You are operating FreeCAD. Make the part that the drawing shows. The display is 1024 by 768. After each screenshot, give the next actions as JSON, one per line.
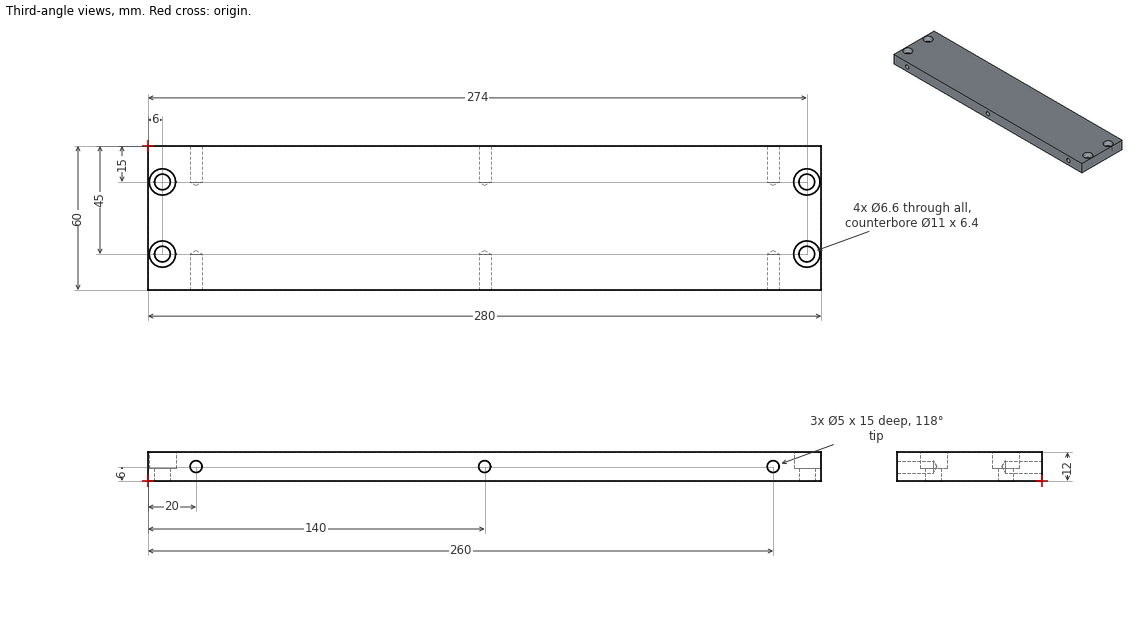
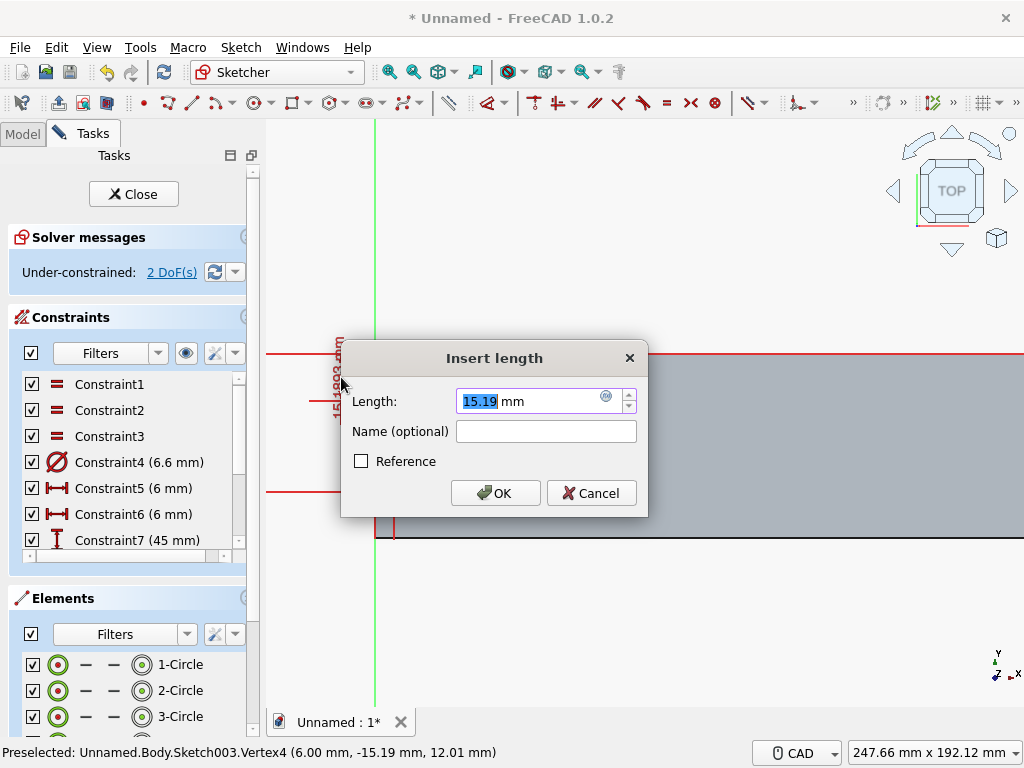
{"action": "type", "text": "15"}
{"action": "key", "text": "Return"}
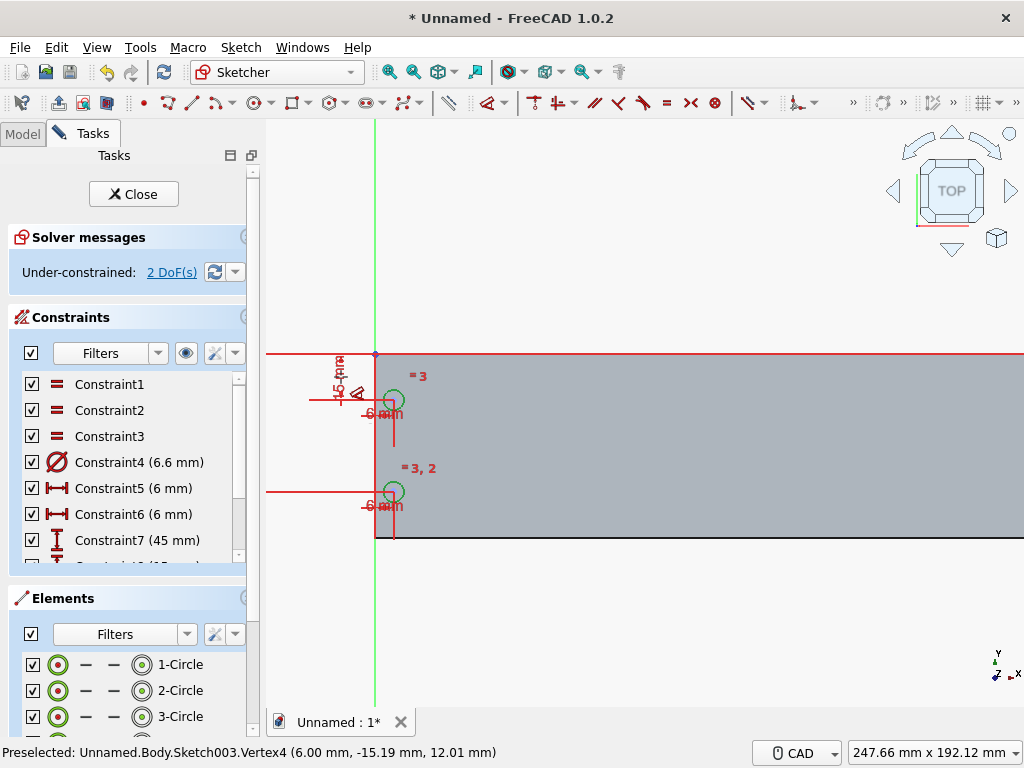
{"action": "scroll", "coordinate": [394, 401], "scroll_direction": "down", "scroll_amount": 4}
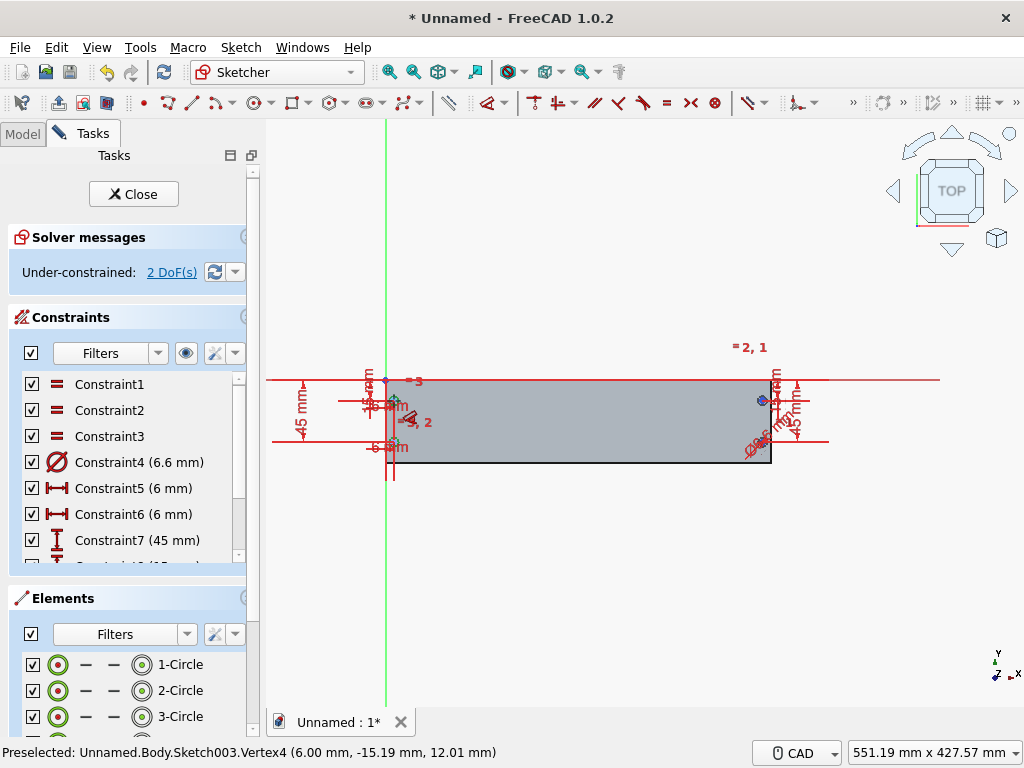
{"action": "left_click", "coordinate": [763, 442]}
{"action": "left_click", "coordinate": [574, 346]}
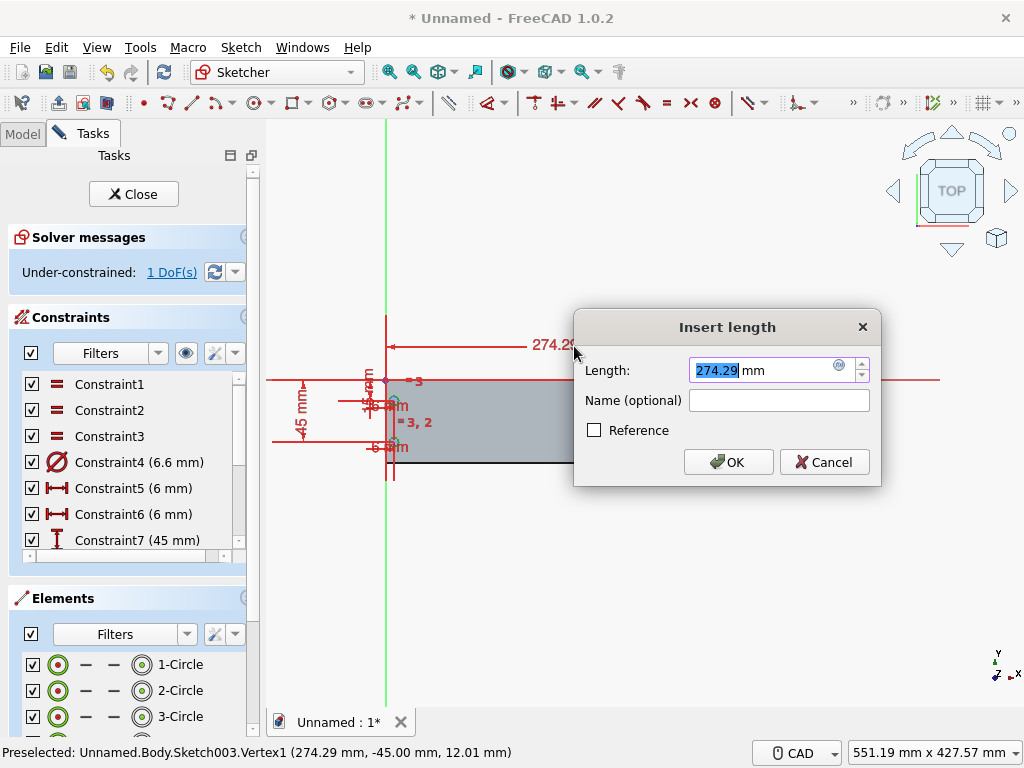
{"action": "type", "text": "274"}
{"action": "key", "text": "Return"}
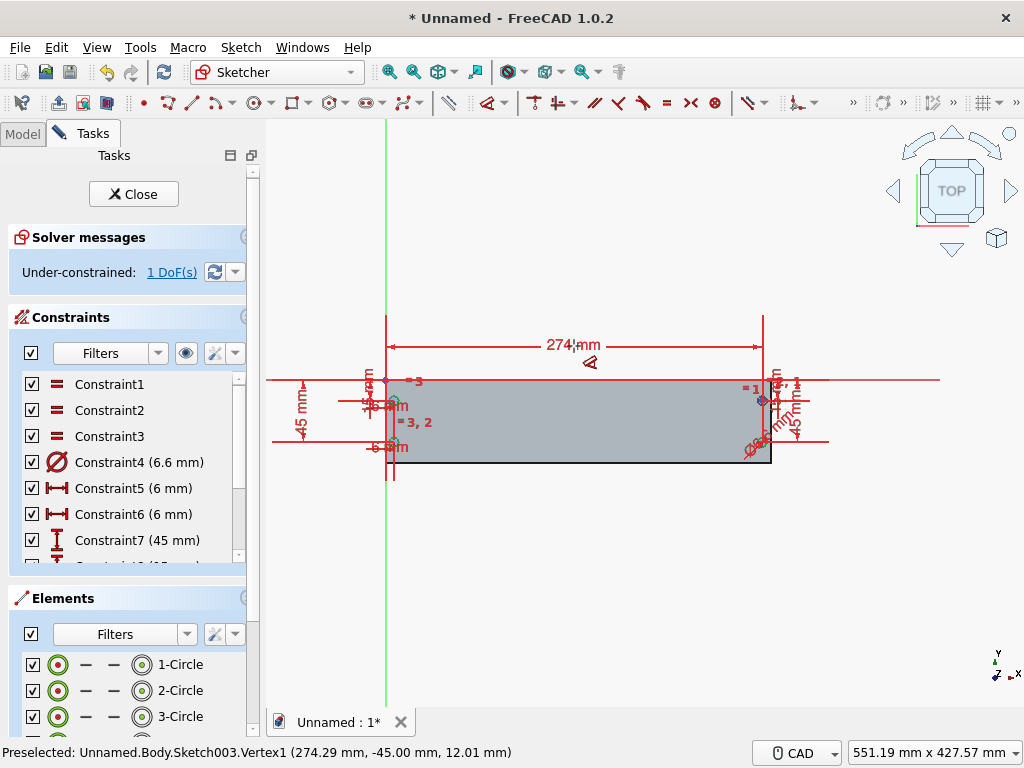
{"action": "left_click", "coordinate": [762, 401]}
{"action": "left_click", "coordinate": [487, 346]}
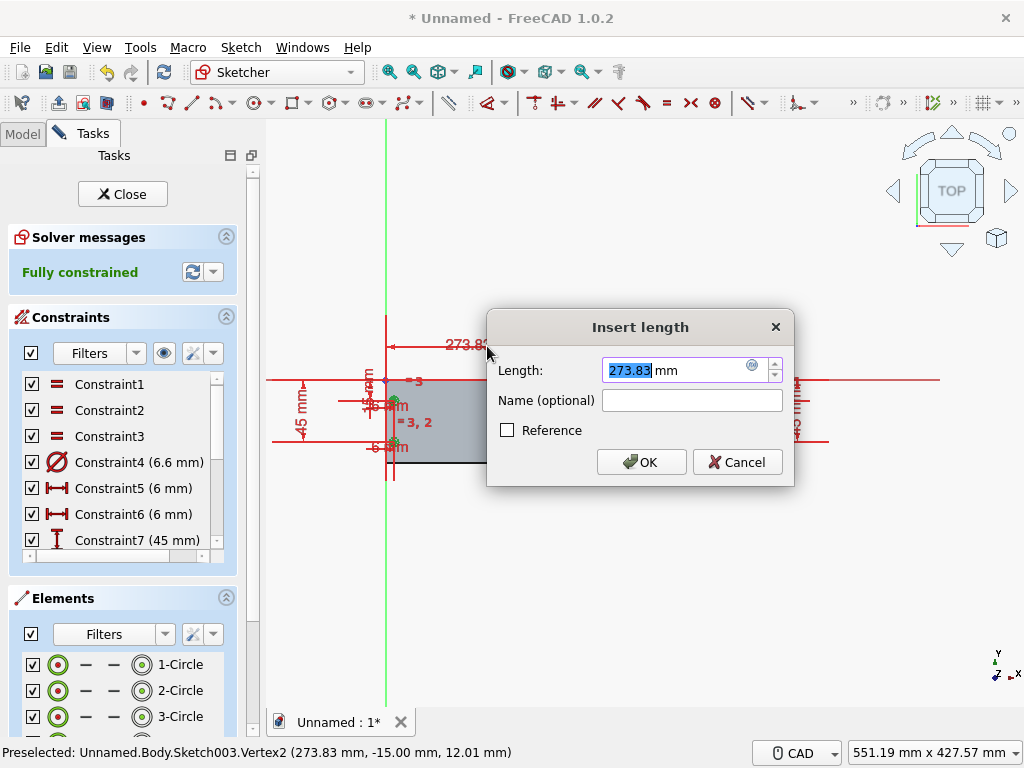
{"action": "type", "text": "274"}
{"action": "key", "text": "Return"}
{"action": "key", "text": "Escape"}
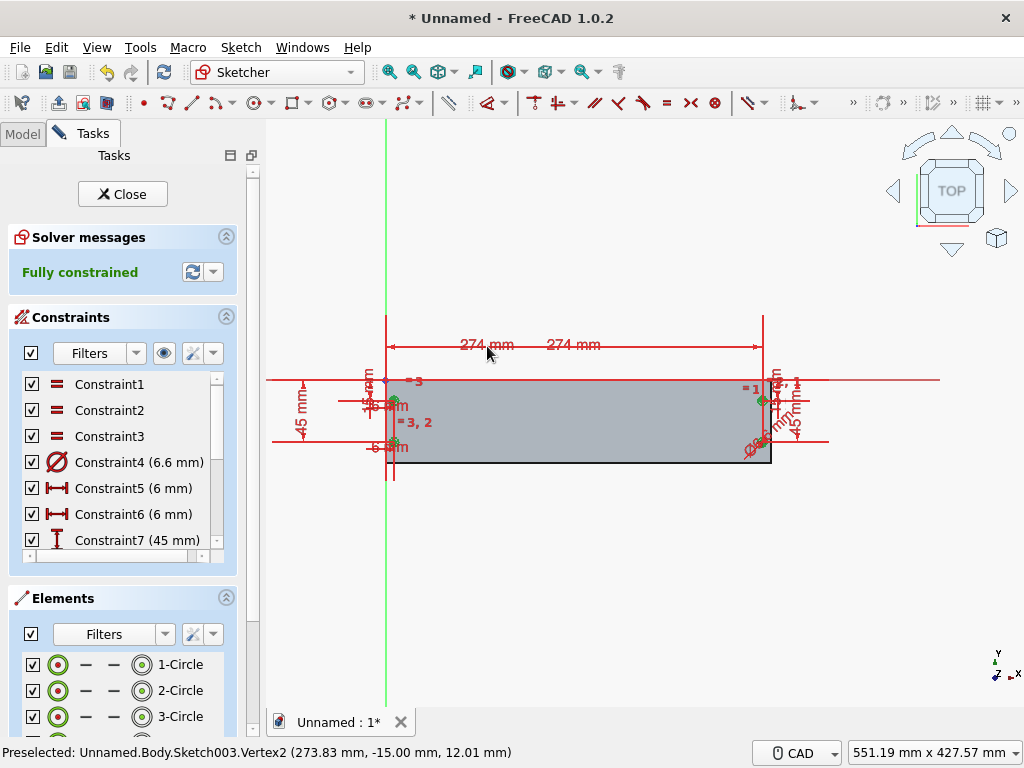
{"action": "left_click", "coordinate": [123, 194]}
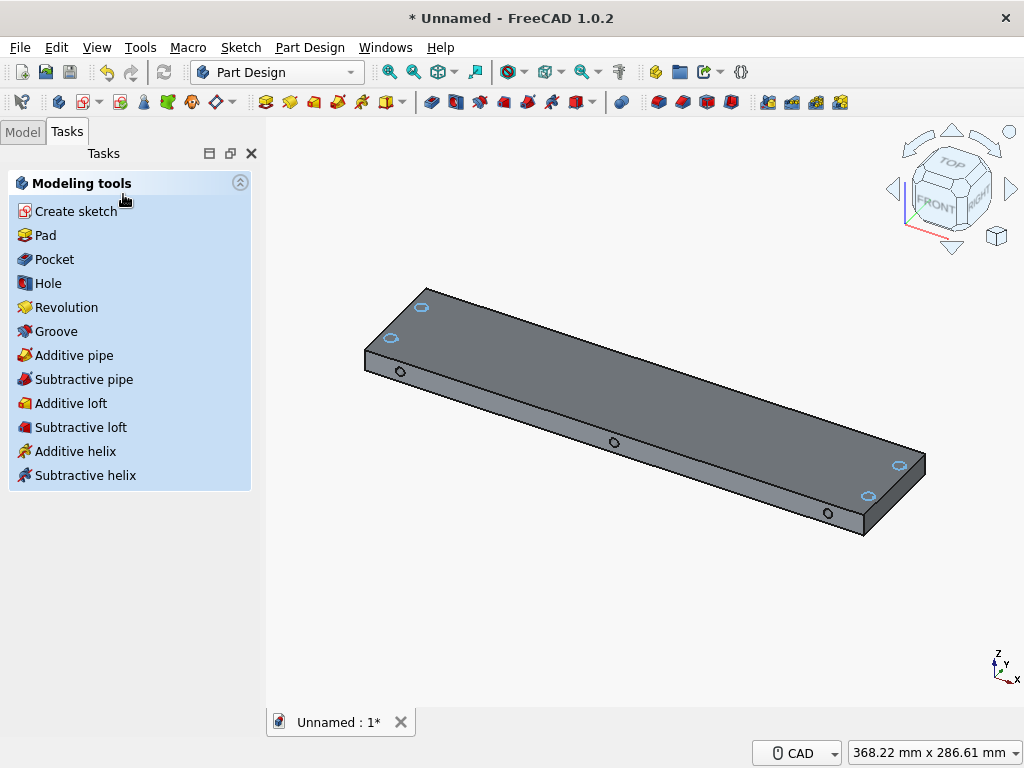
{"action": "left_click", "coordinate": [456, 102]}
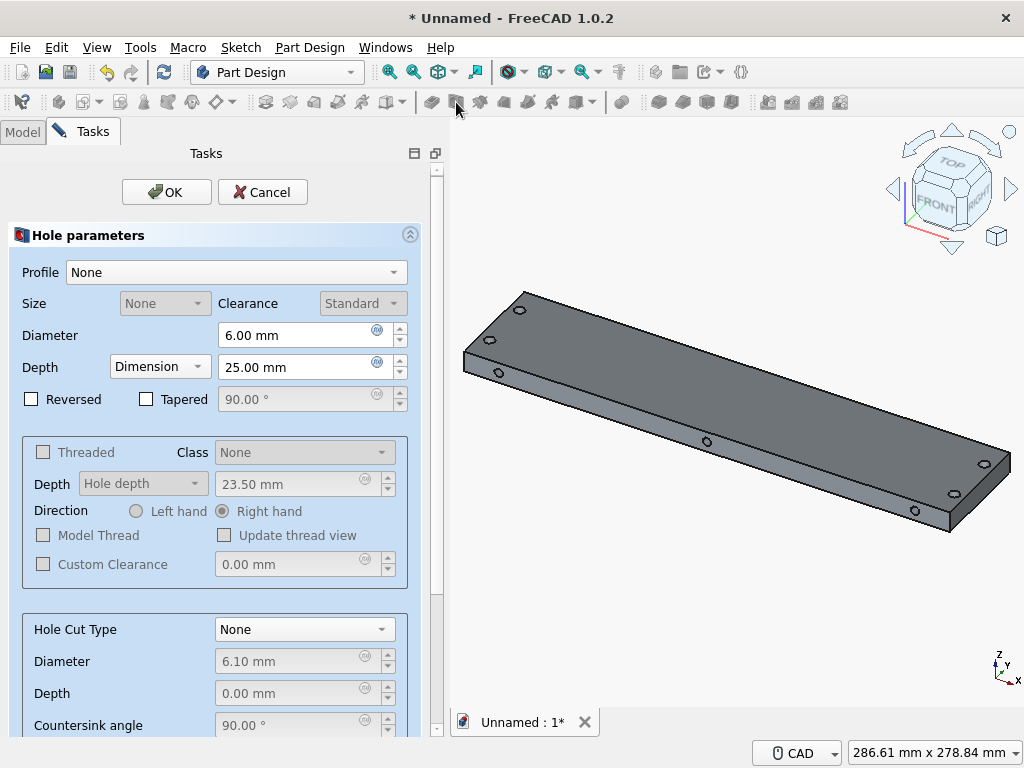
{"action": "triple_click", "coordinate": [305, 335]}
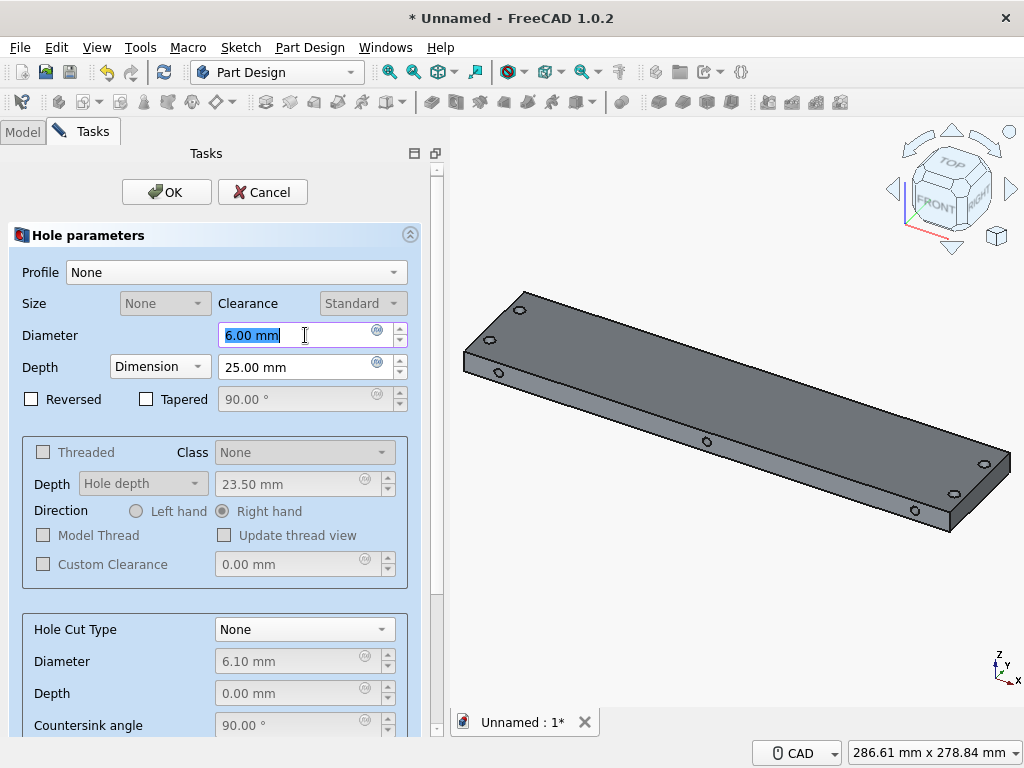
{"action": "type", "text": "6.6"}
{"action": "key", "text": "Tab"}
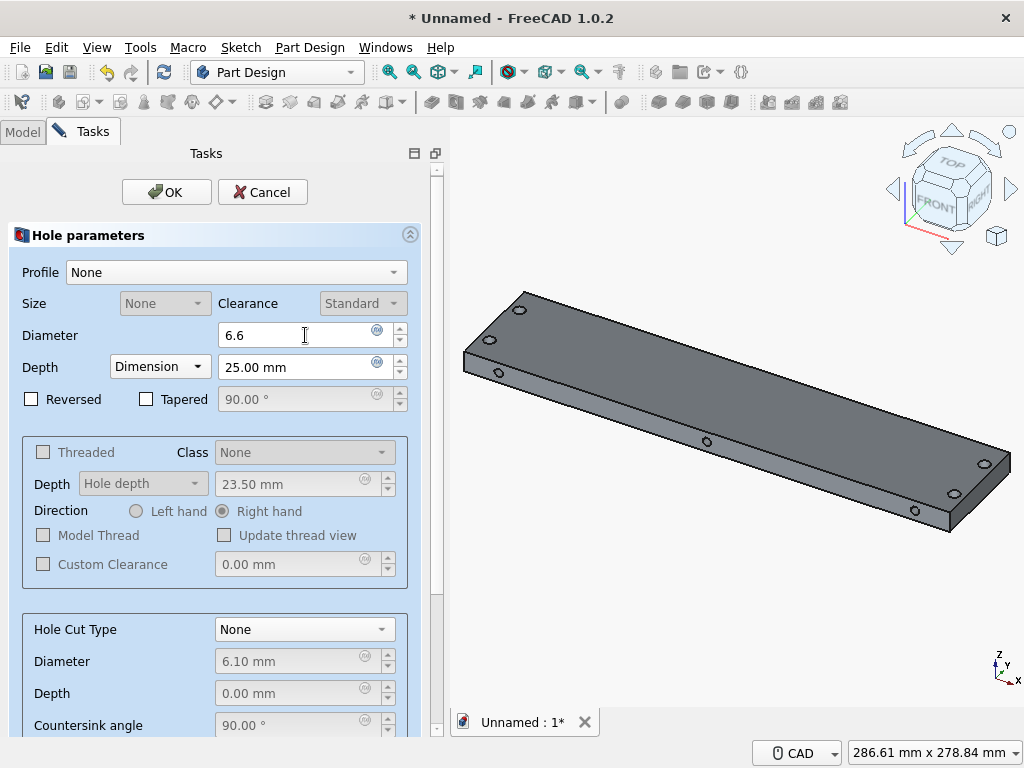
{"action": "left_click", "coordinate": [161, 366]}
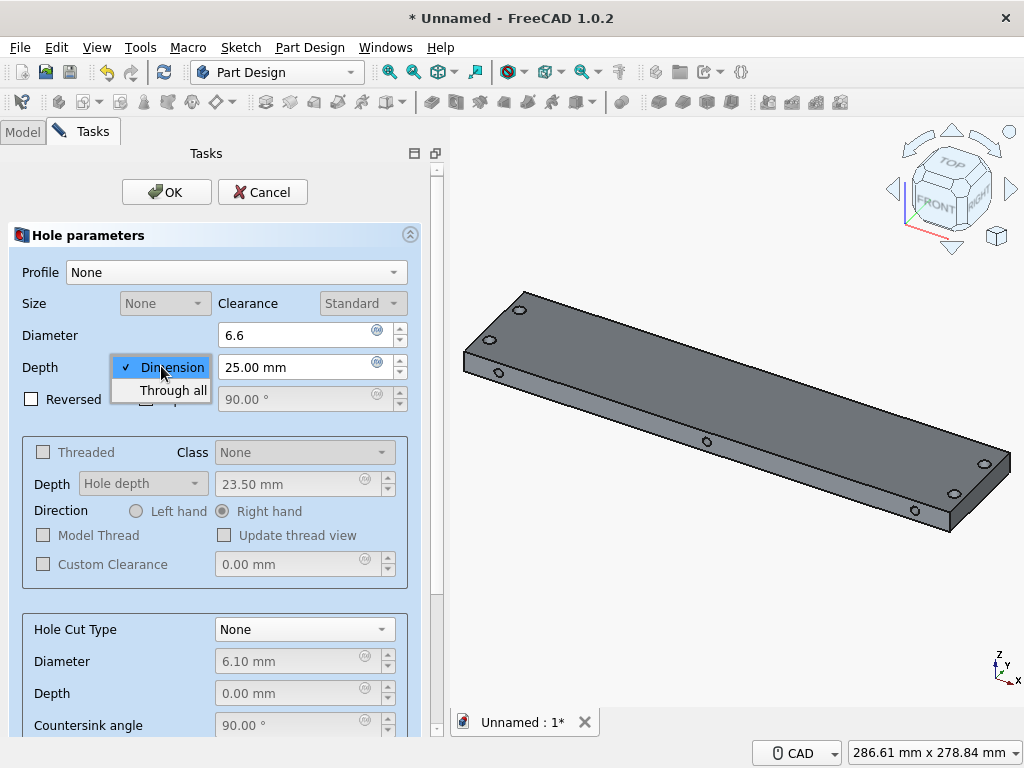
{"action": "left_click", "coordinate": [160, 390]}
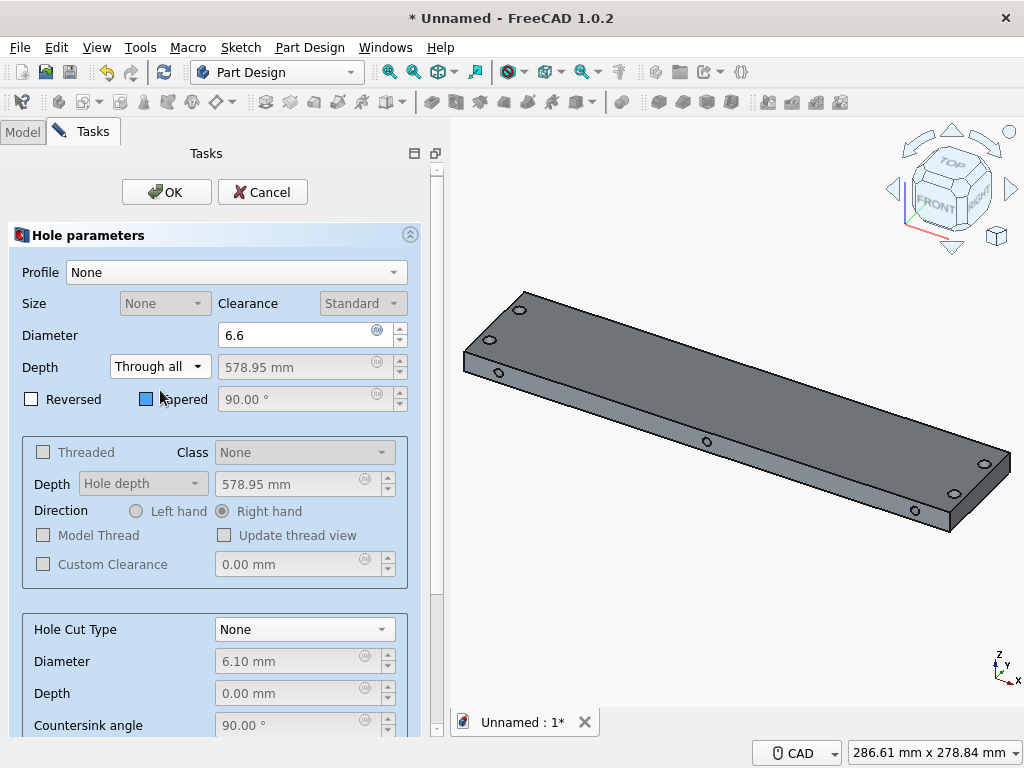
{"action": "left_click", "coordinate": [306, 630]}